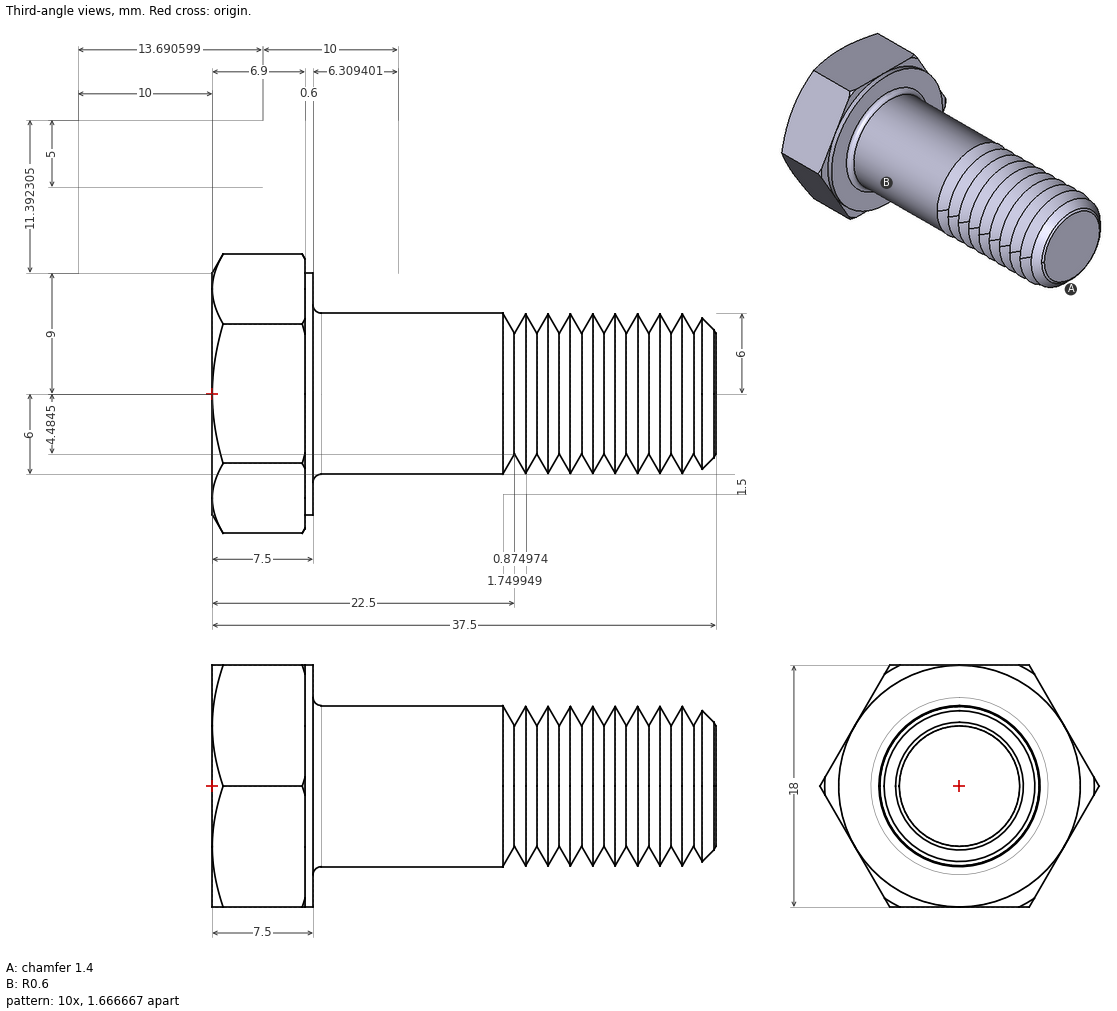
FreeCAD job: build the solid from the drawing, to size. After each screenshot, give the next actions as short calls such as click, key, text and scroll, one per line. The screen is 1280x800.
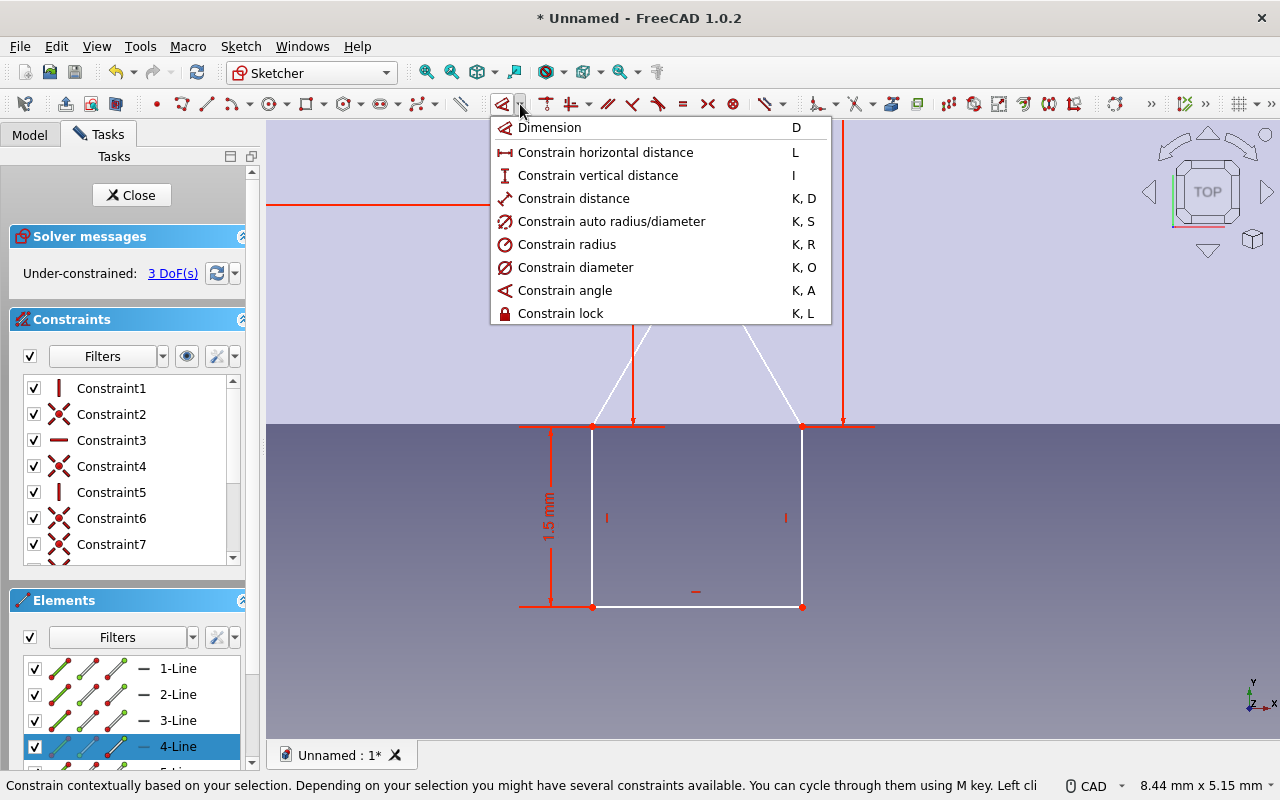
click(661, 176)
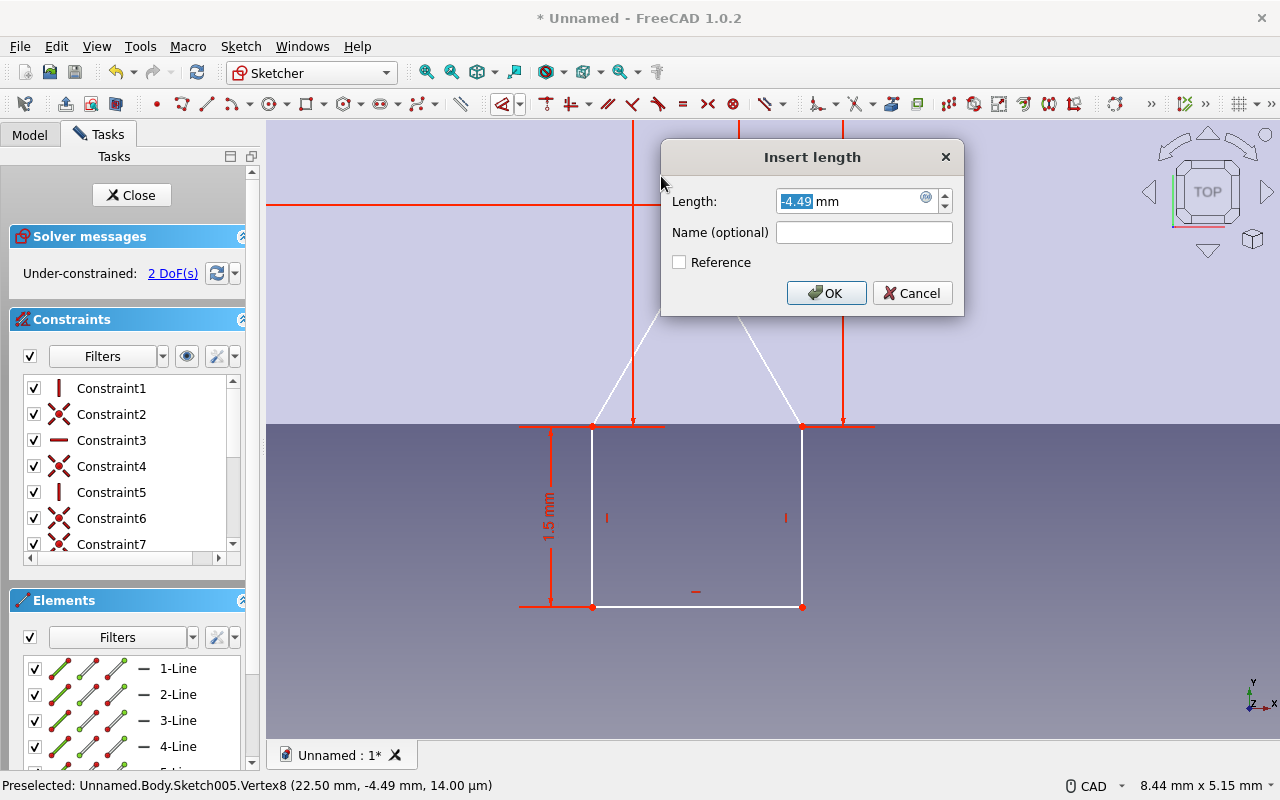
text(-4.4845)
key(Return)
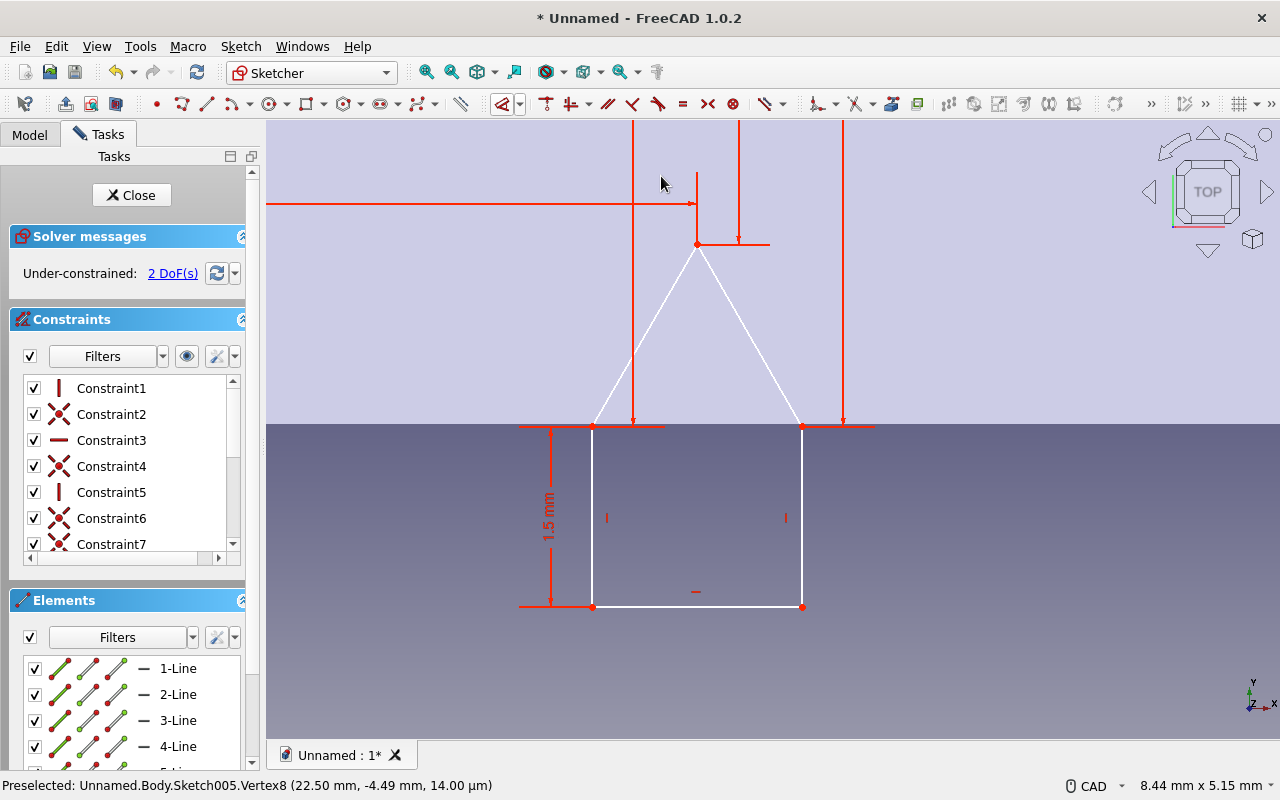
click(655, 607)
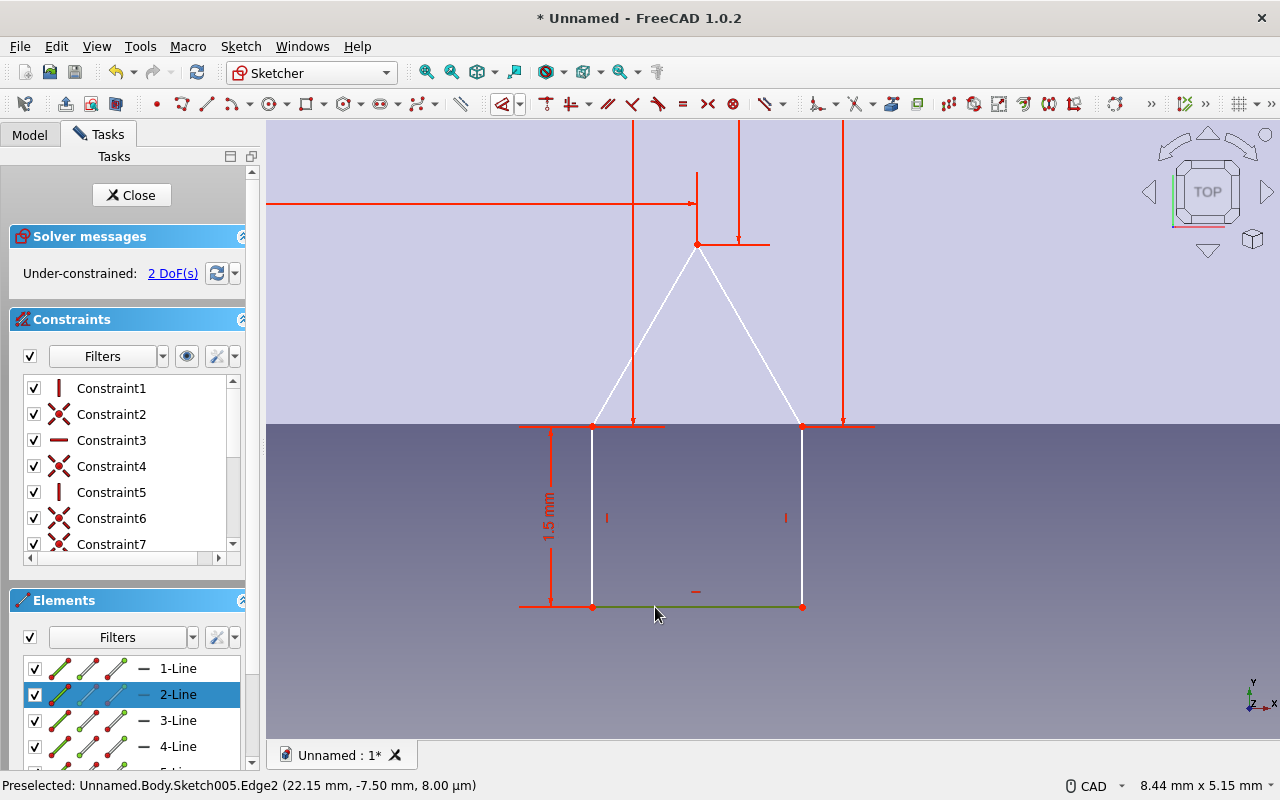
click(520, 104)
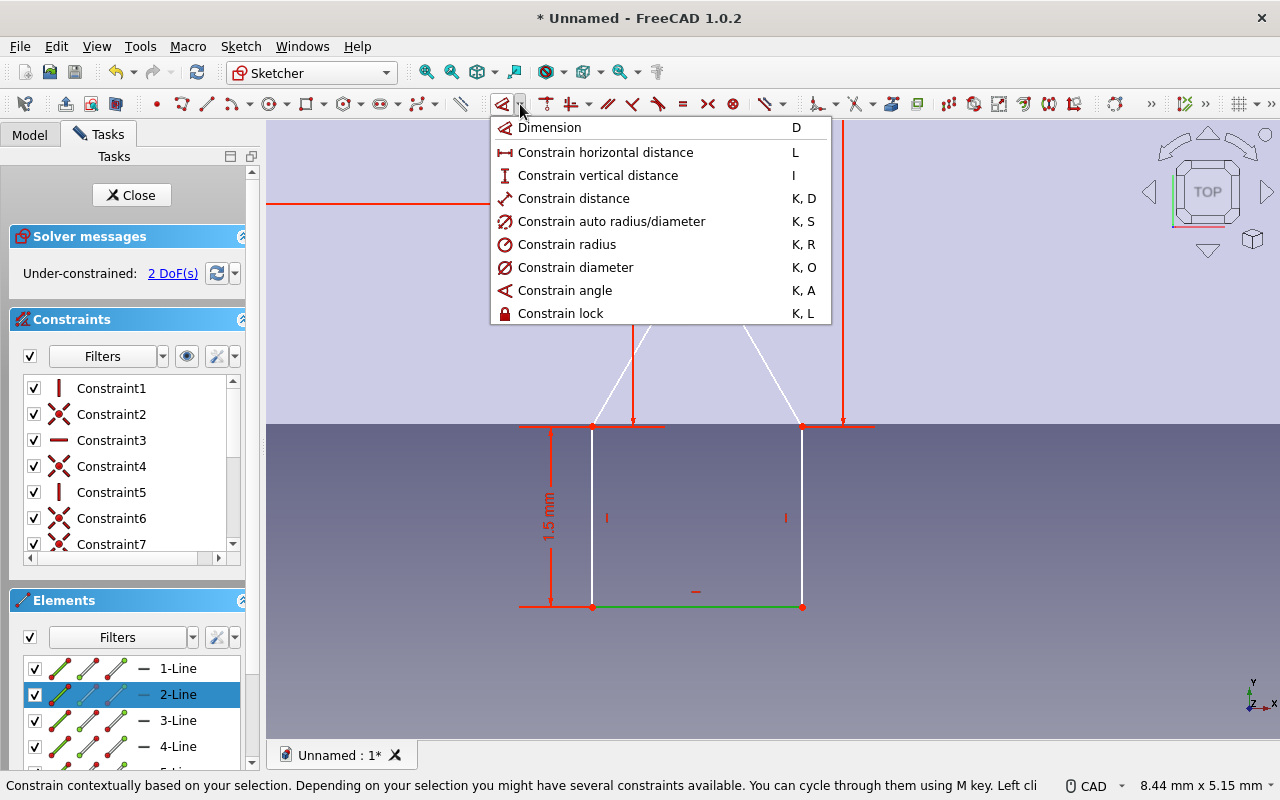
click(661, 152)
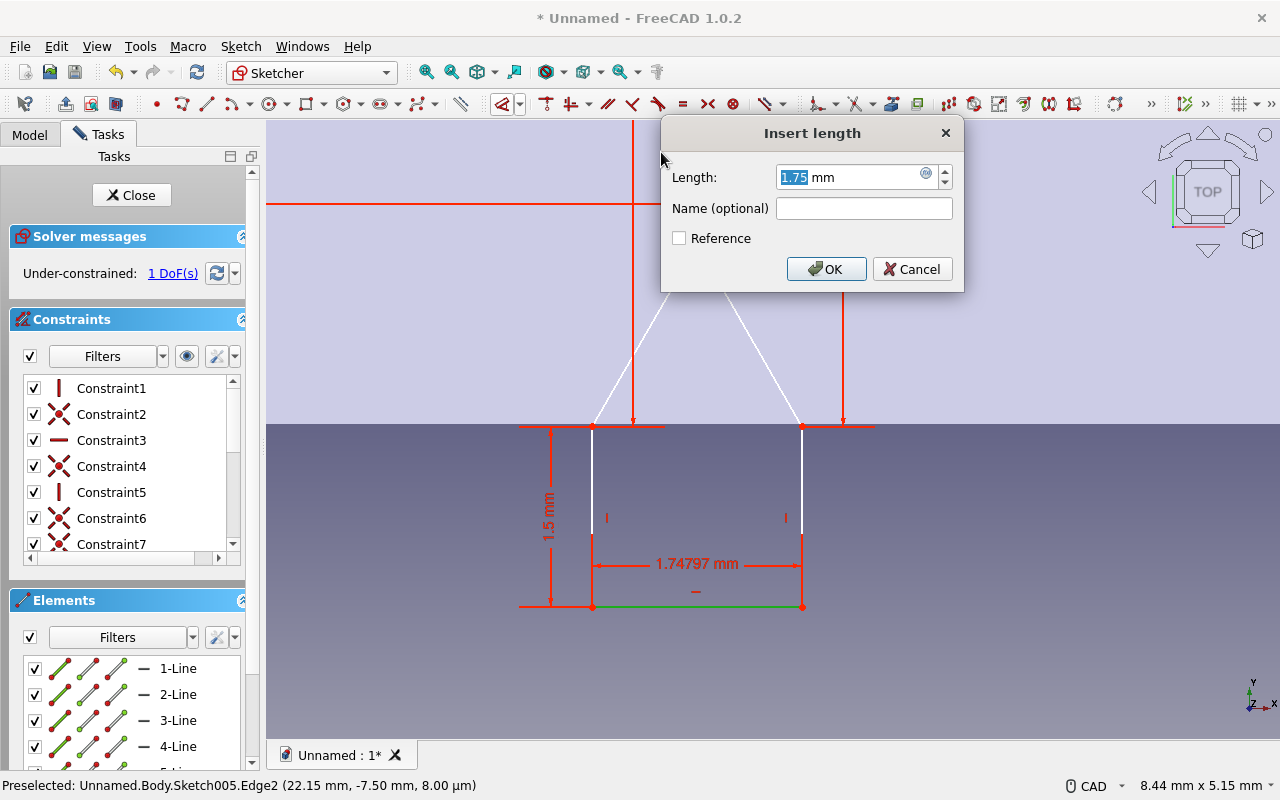
text(1.749949)
key(Return)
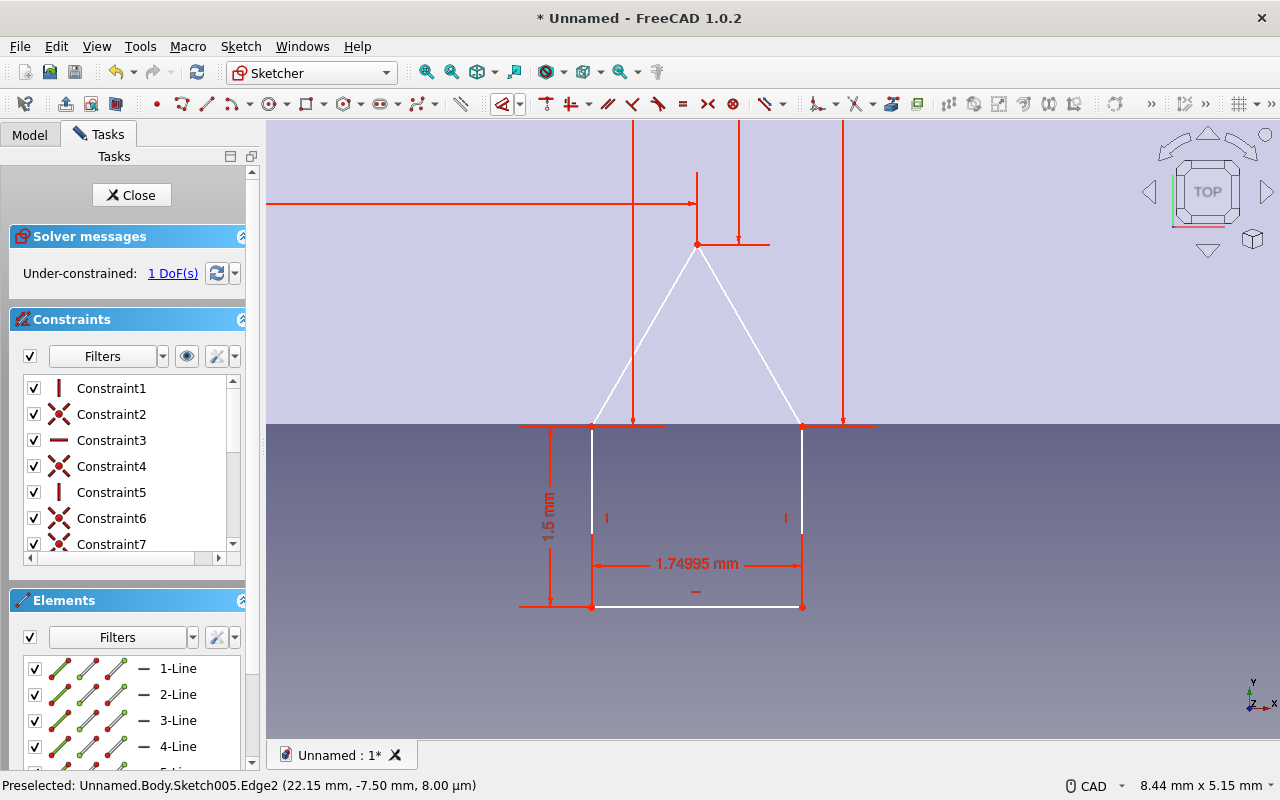
click(771, 372)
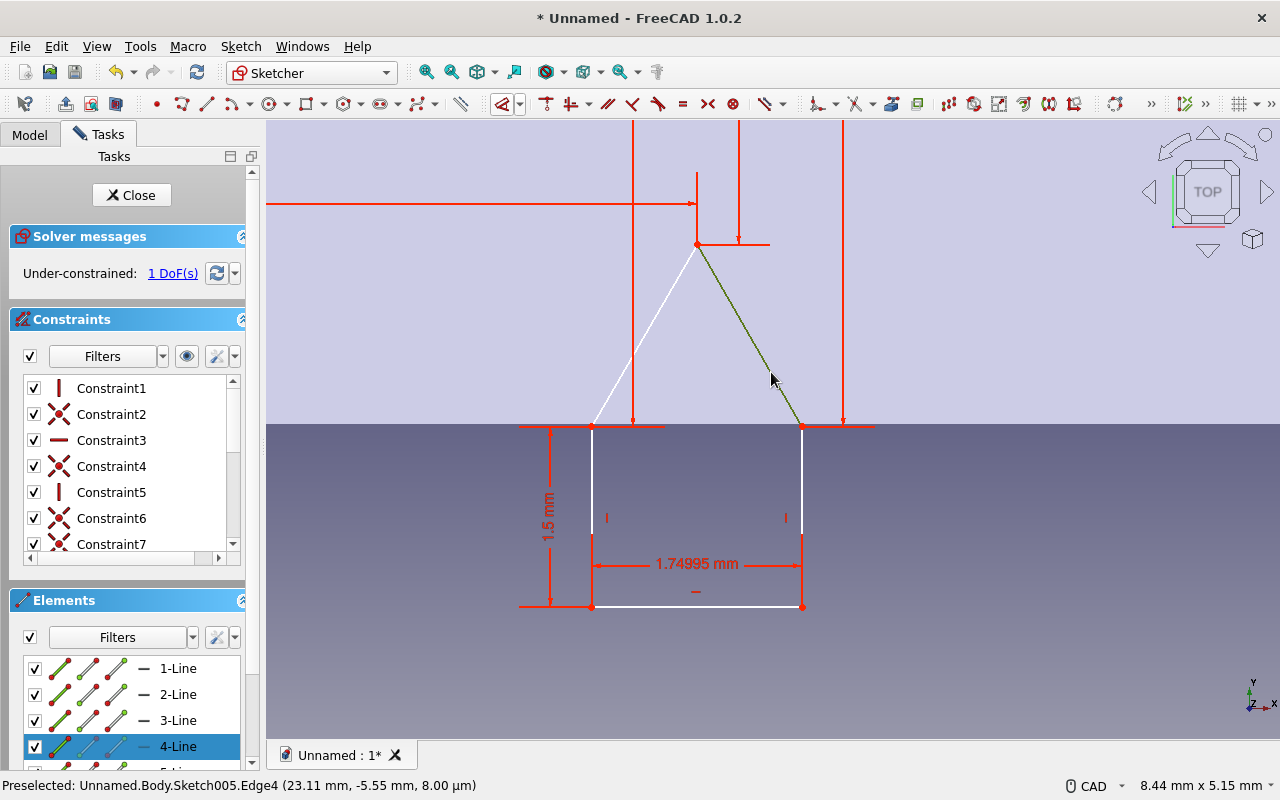
click(520, 104)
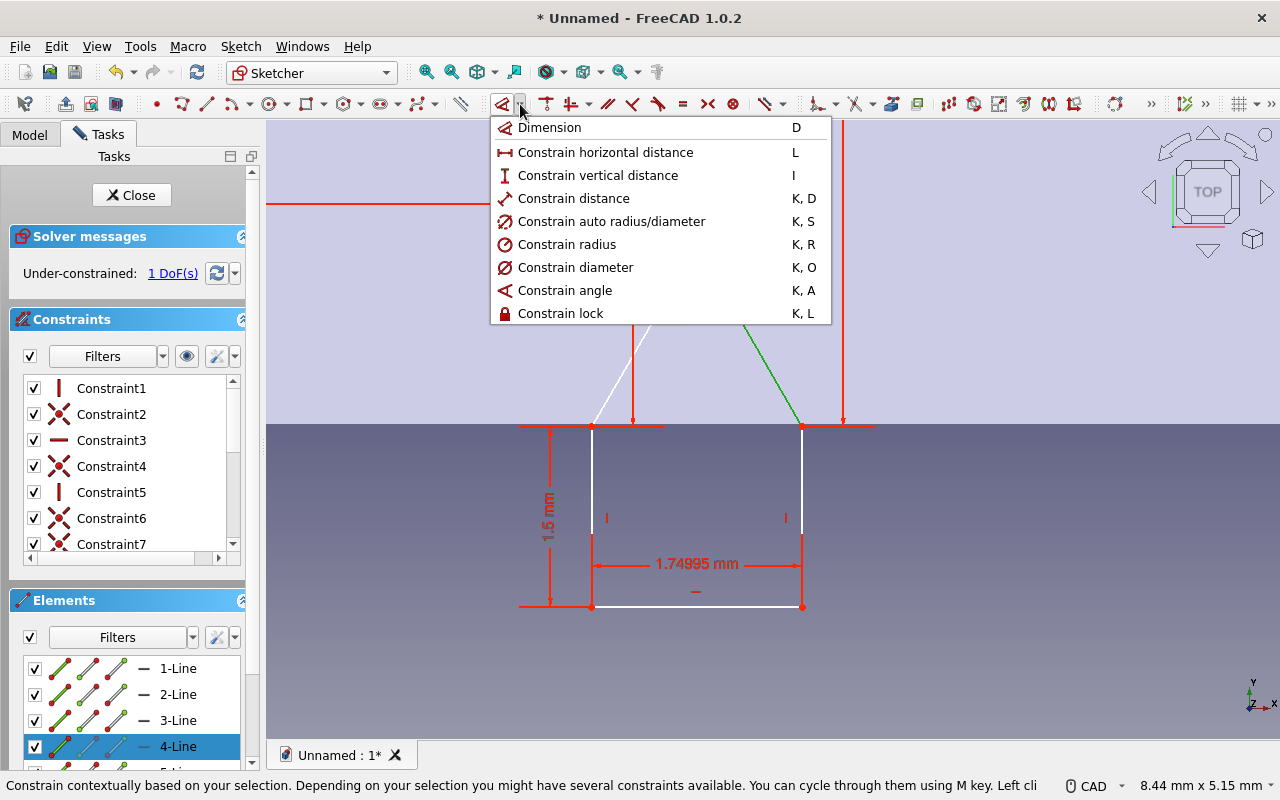
click(661, 152)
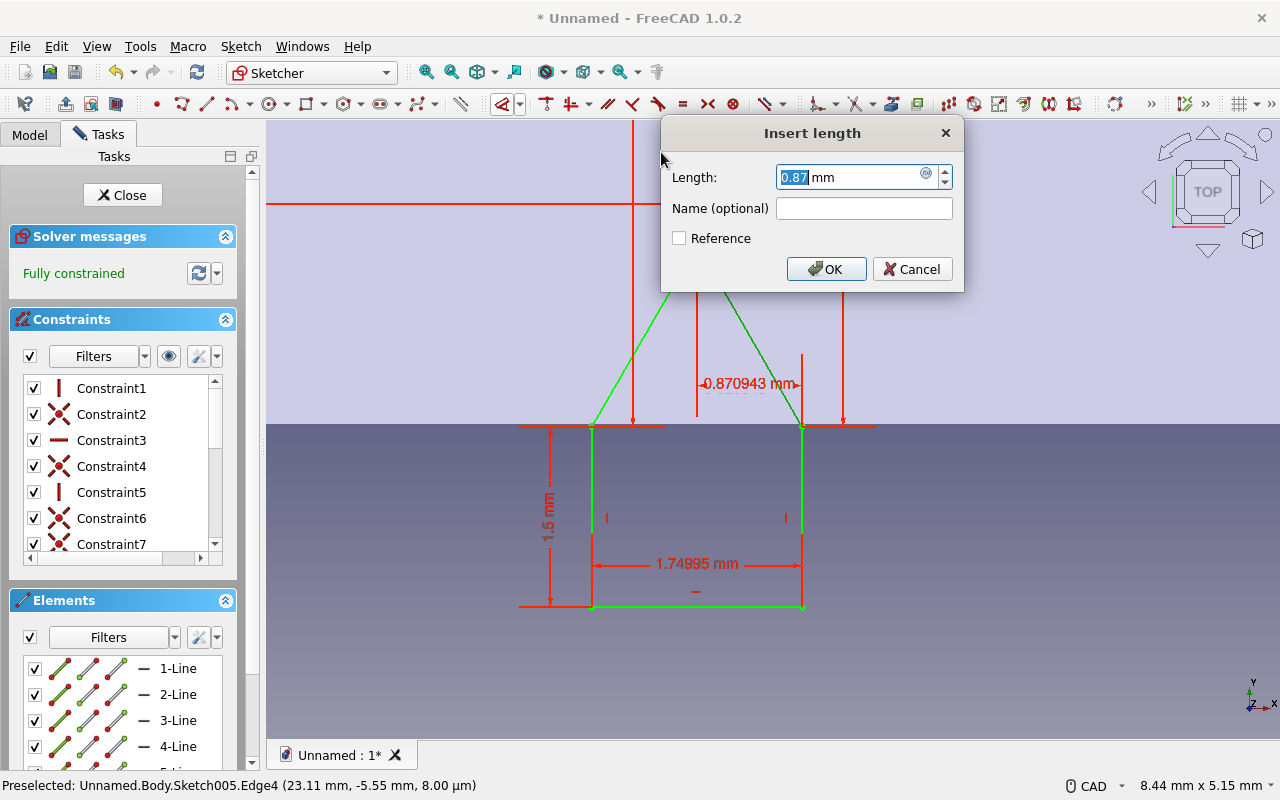
text(0.874974)
key(Return)